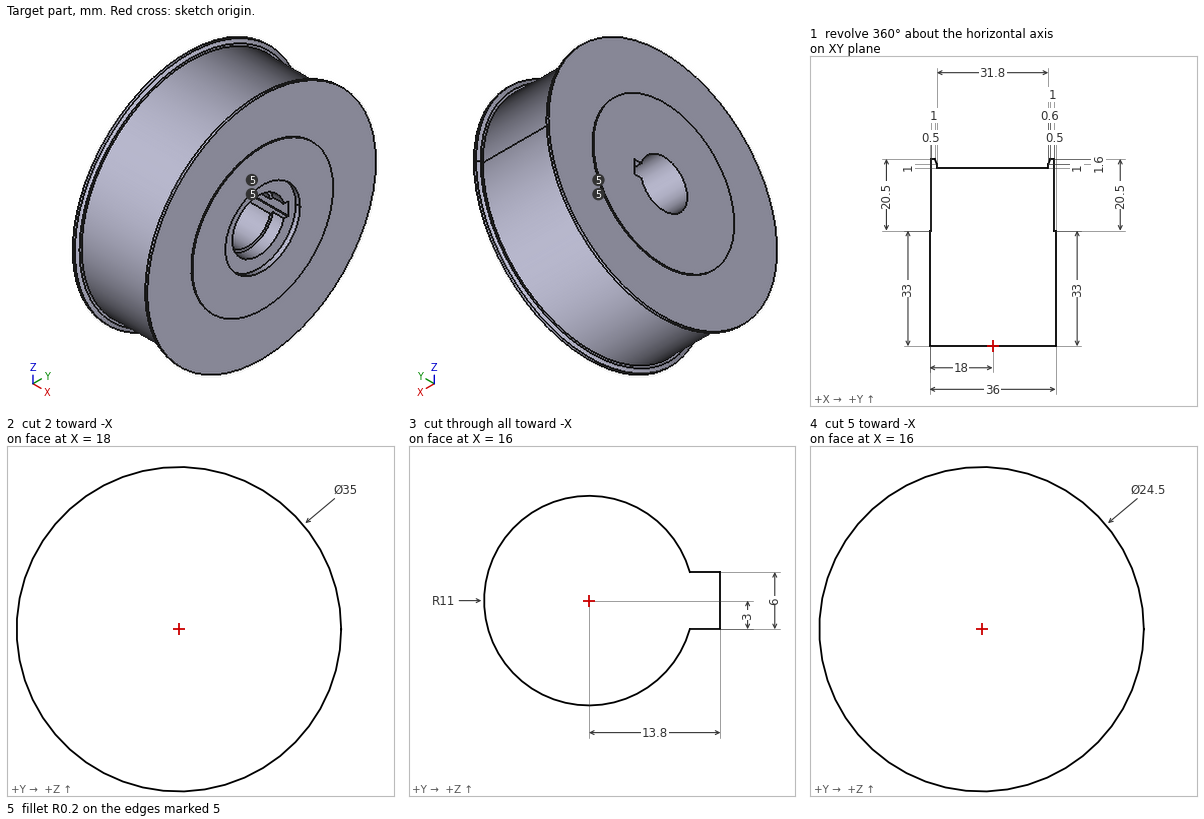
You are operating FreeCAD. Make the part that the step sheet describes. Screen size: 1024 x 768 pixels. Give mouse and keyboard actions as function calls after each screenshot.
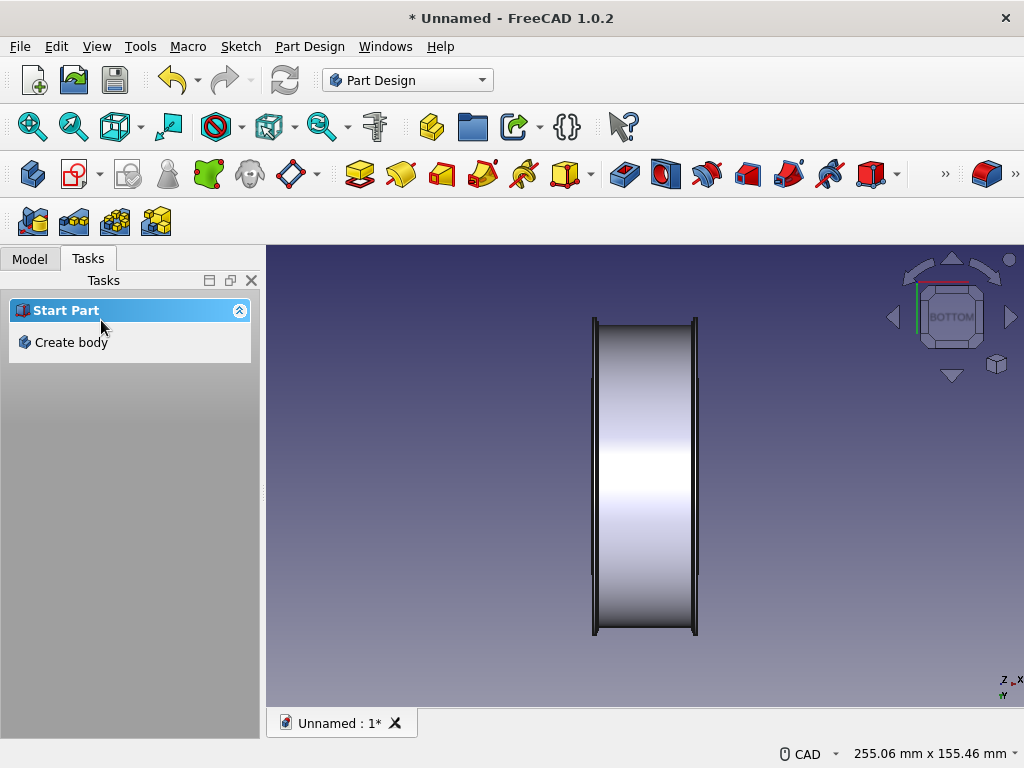
key(0)